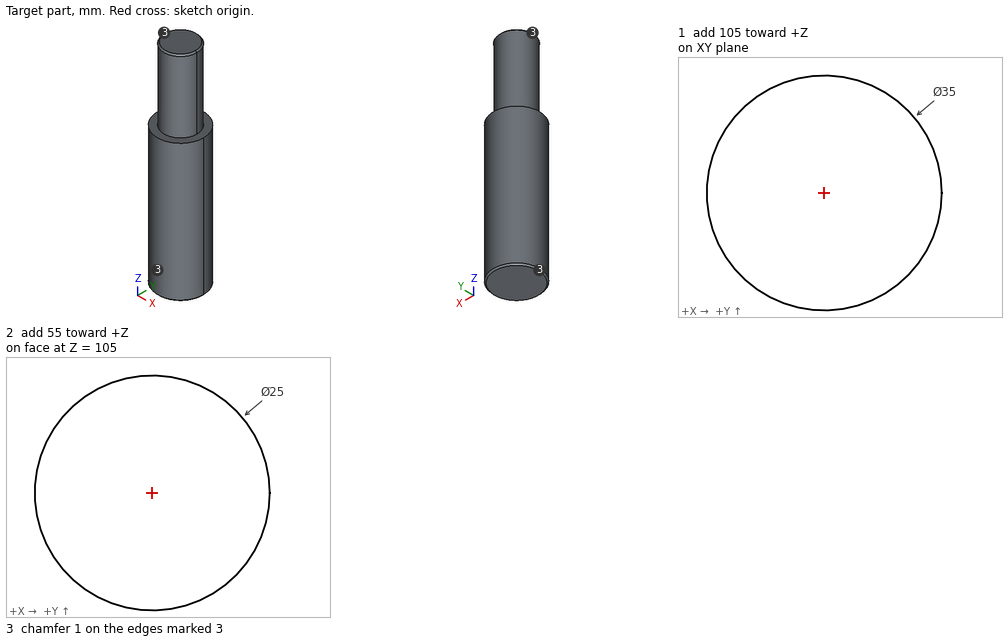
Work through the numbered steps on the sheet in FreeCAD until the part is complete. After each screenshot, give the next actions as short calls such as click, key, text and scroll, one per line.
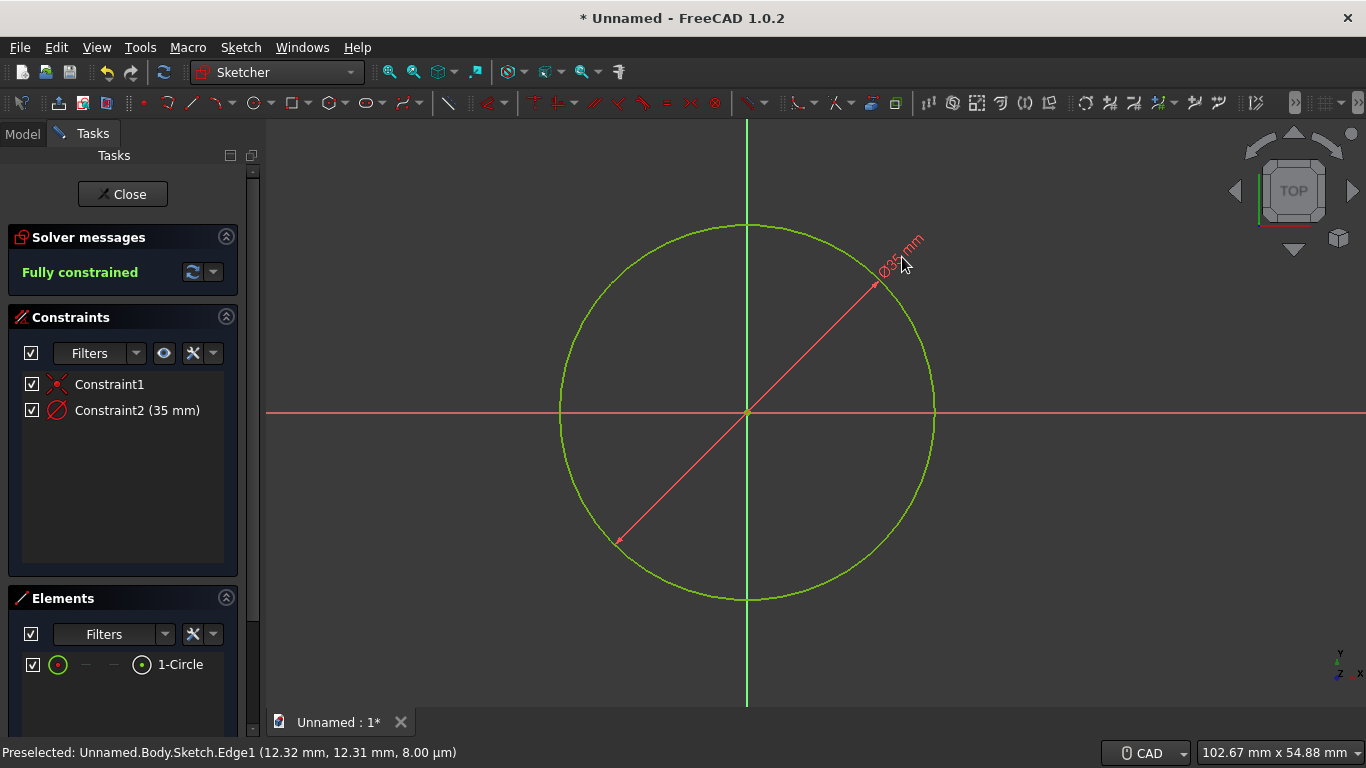
click(123, 194)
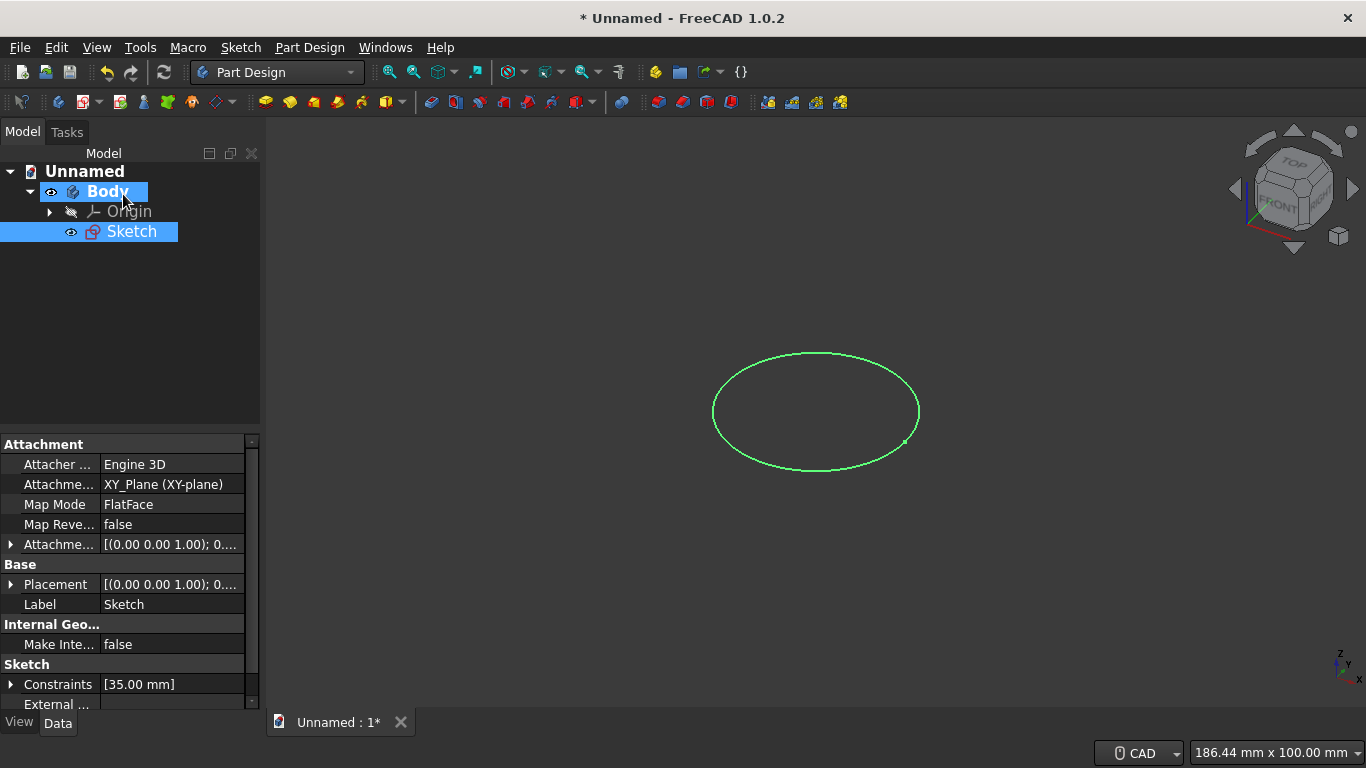
click(266, 102)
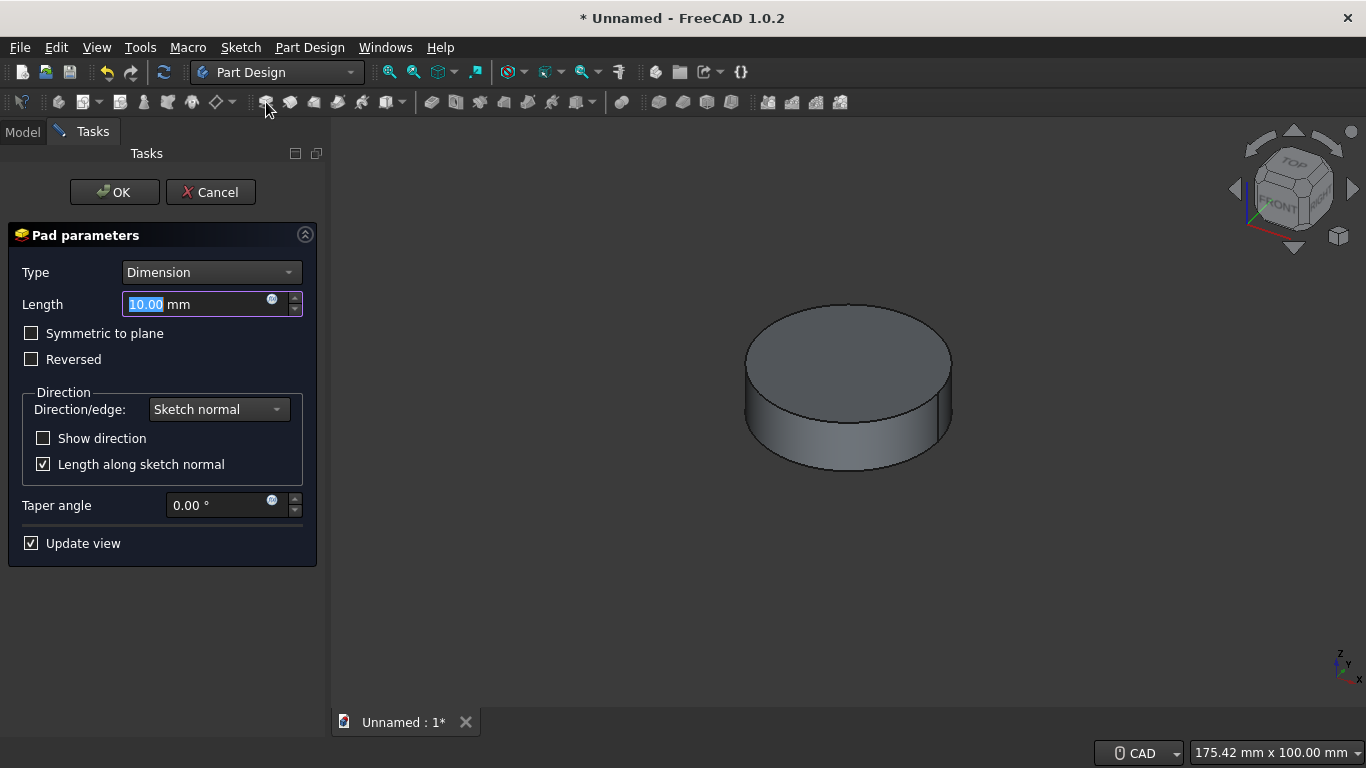
text(105)
key(Tab)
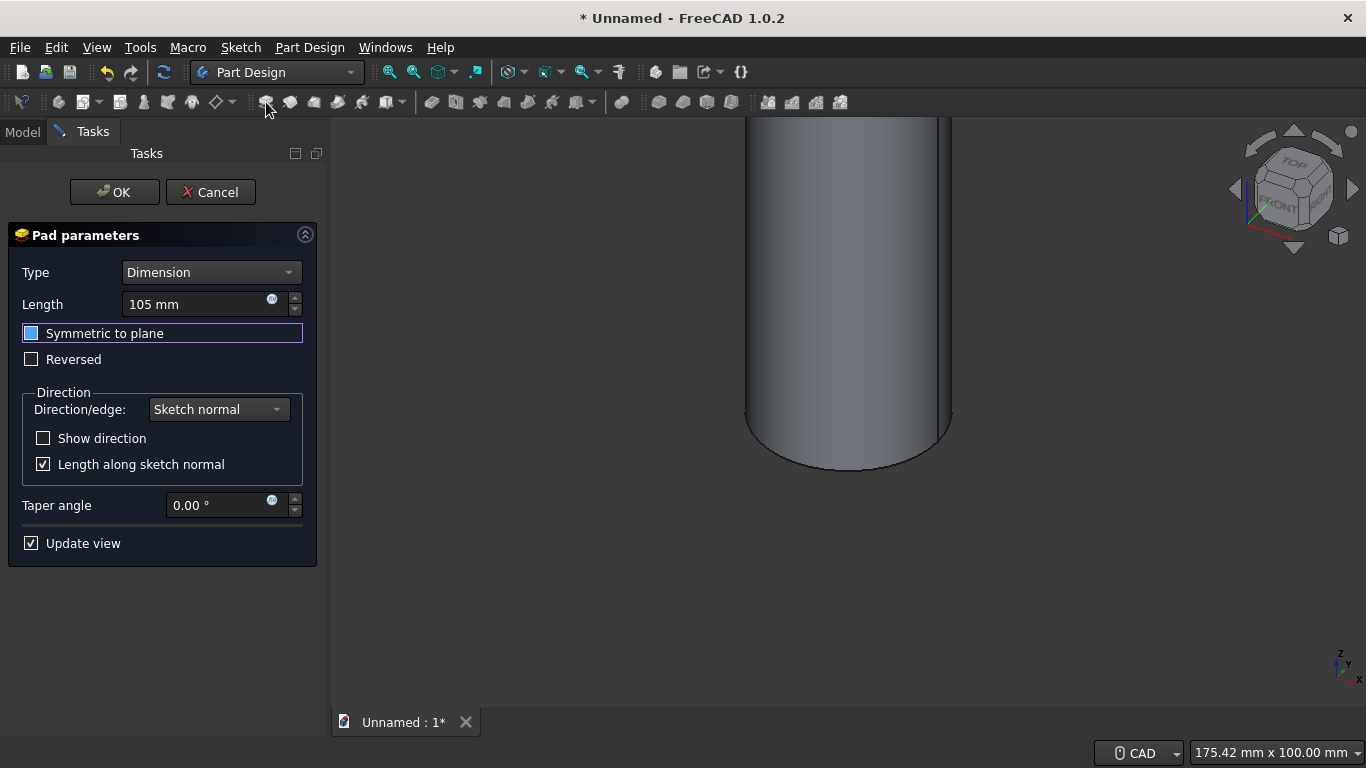
click(115, 192)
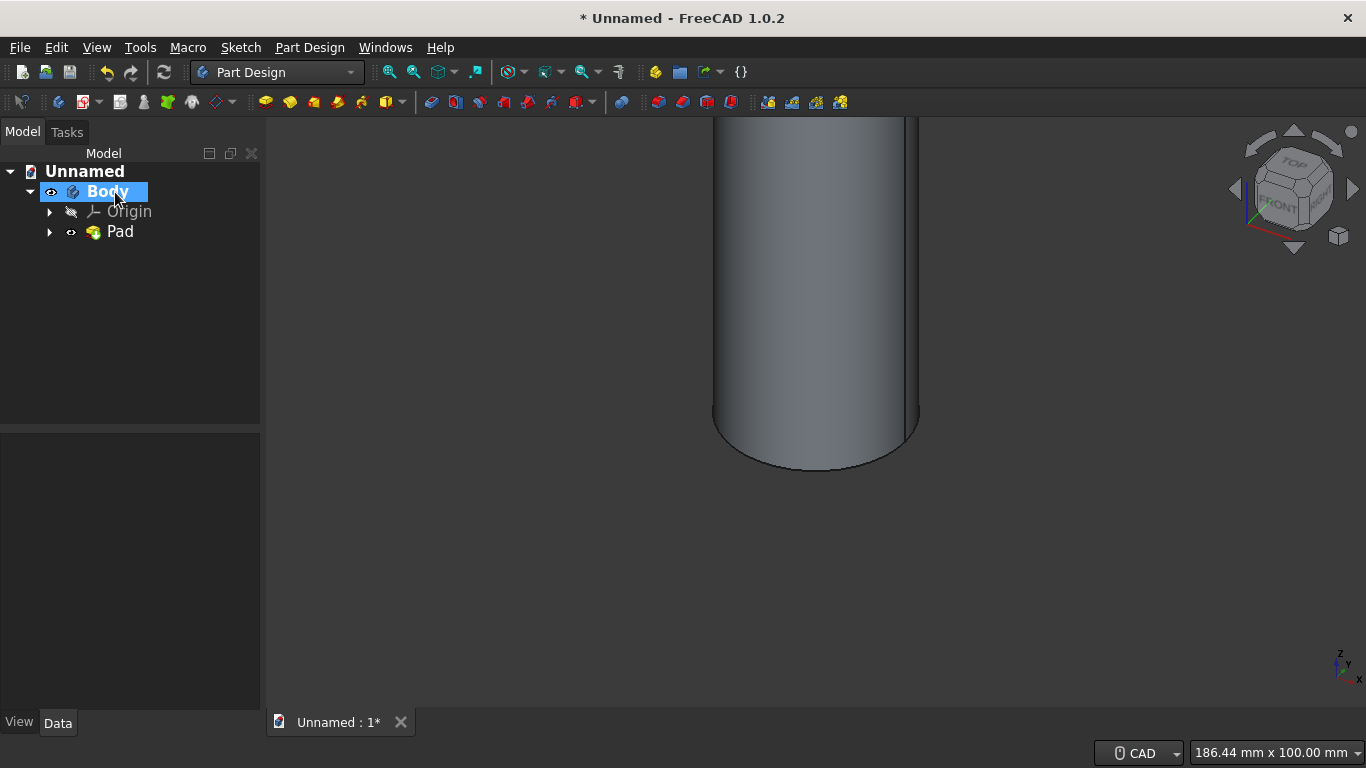
click(390, 72)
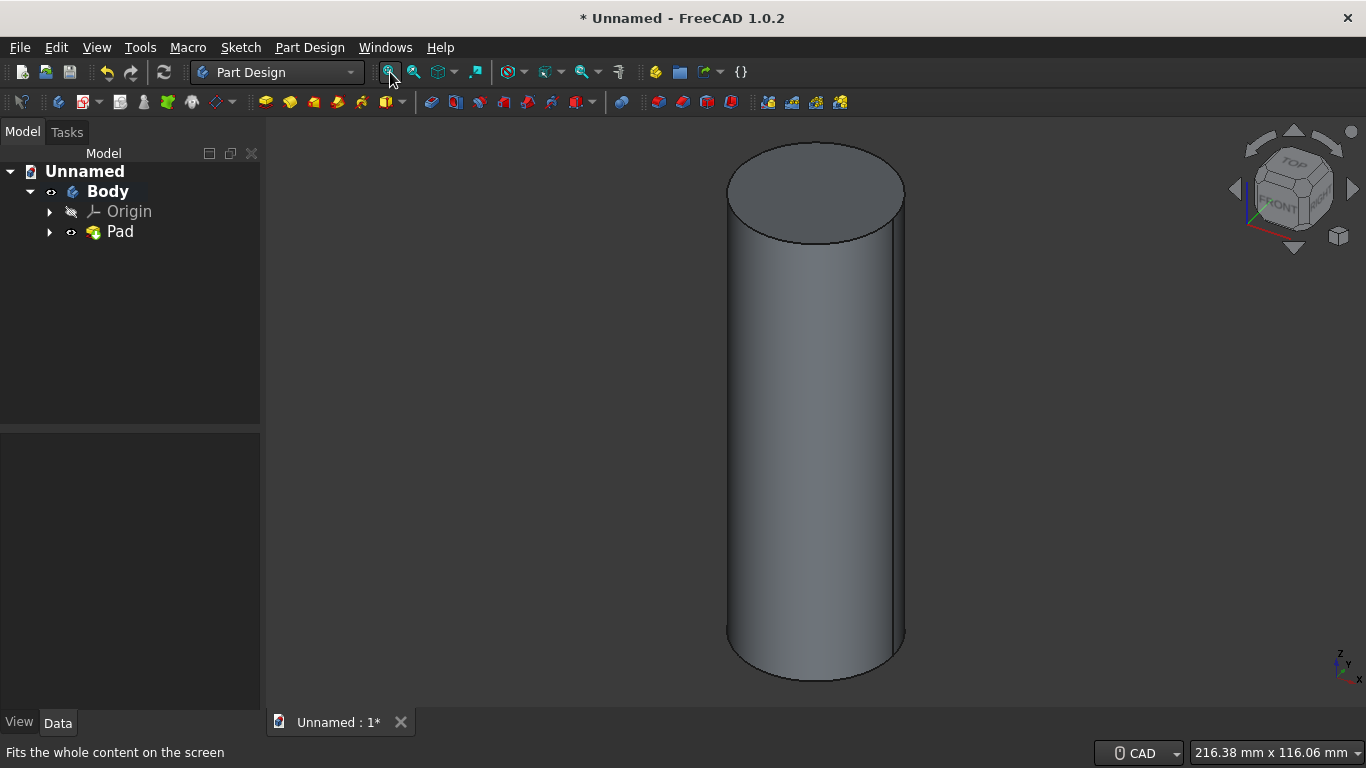
click(816, 192)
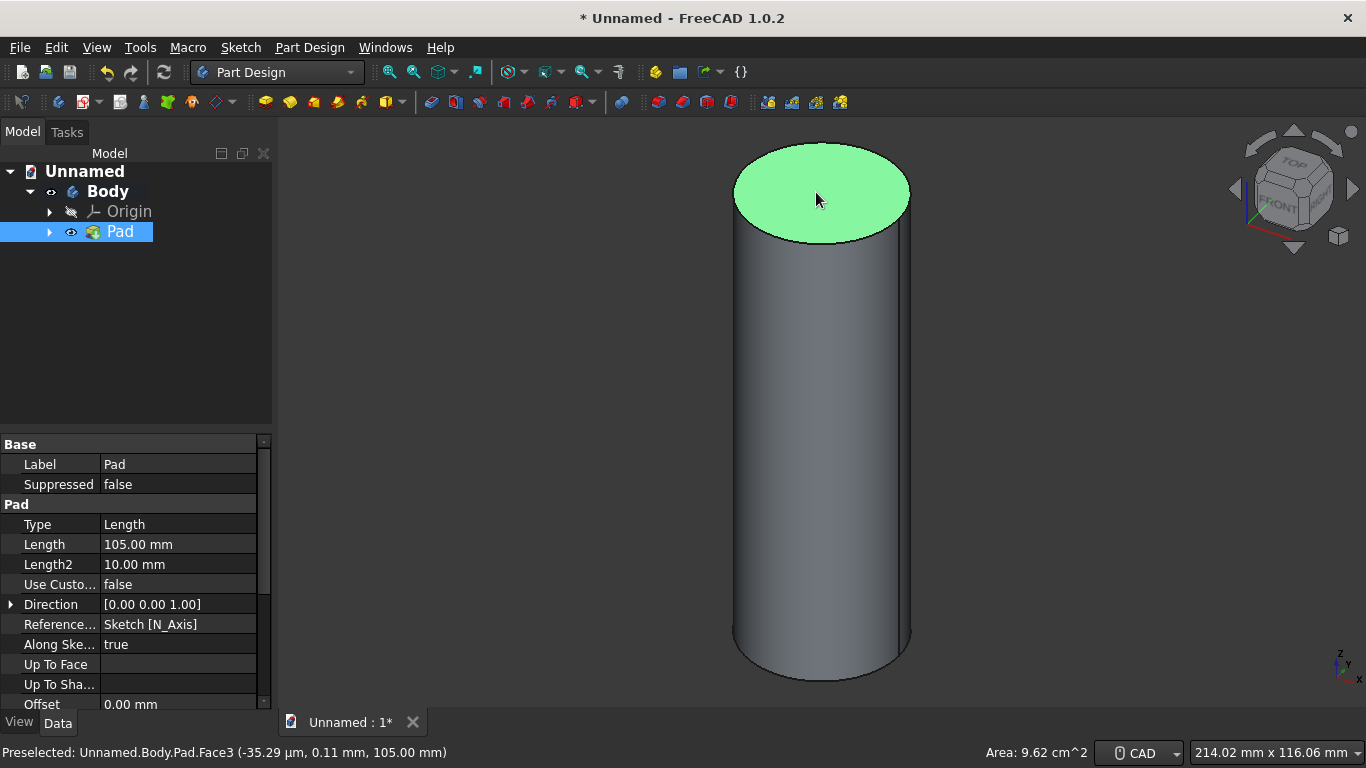
click(84, 102)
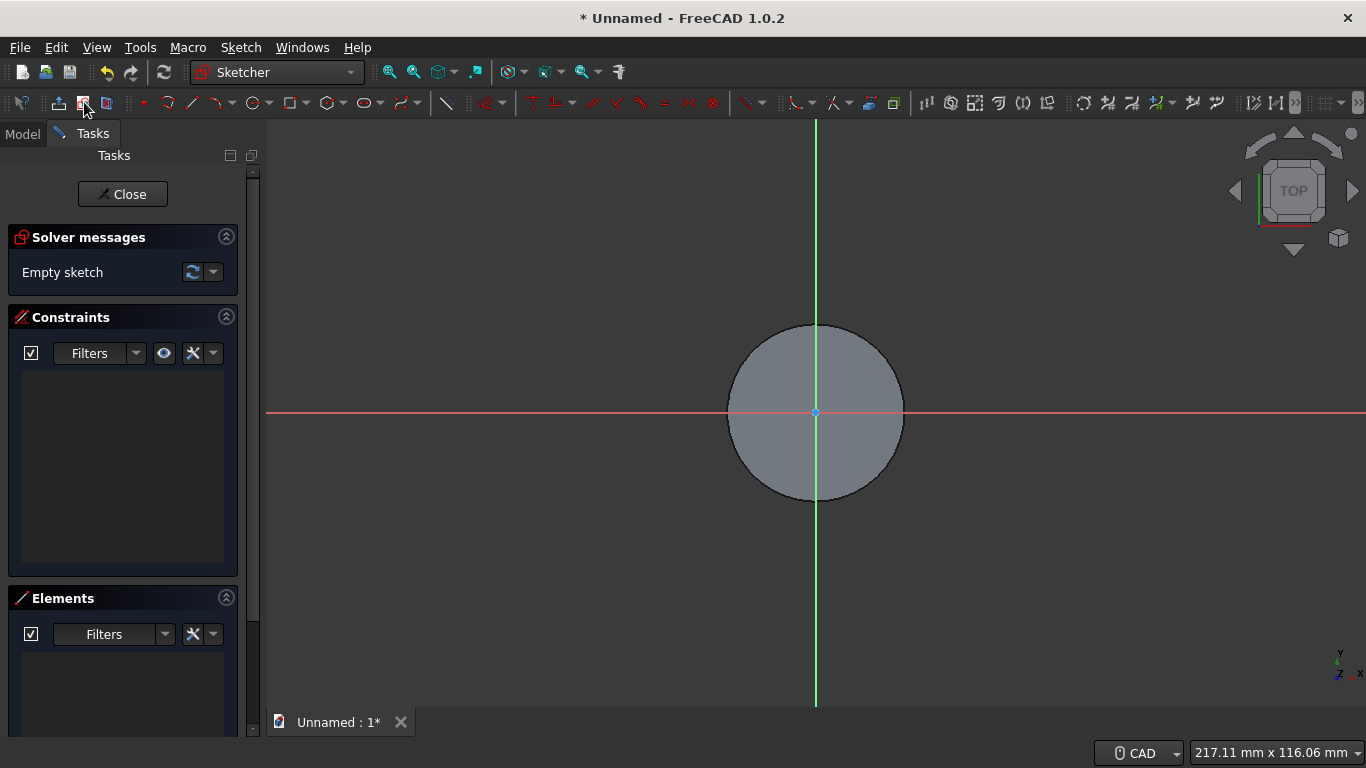
scroll(856, 413, up, 5)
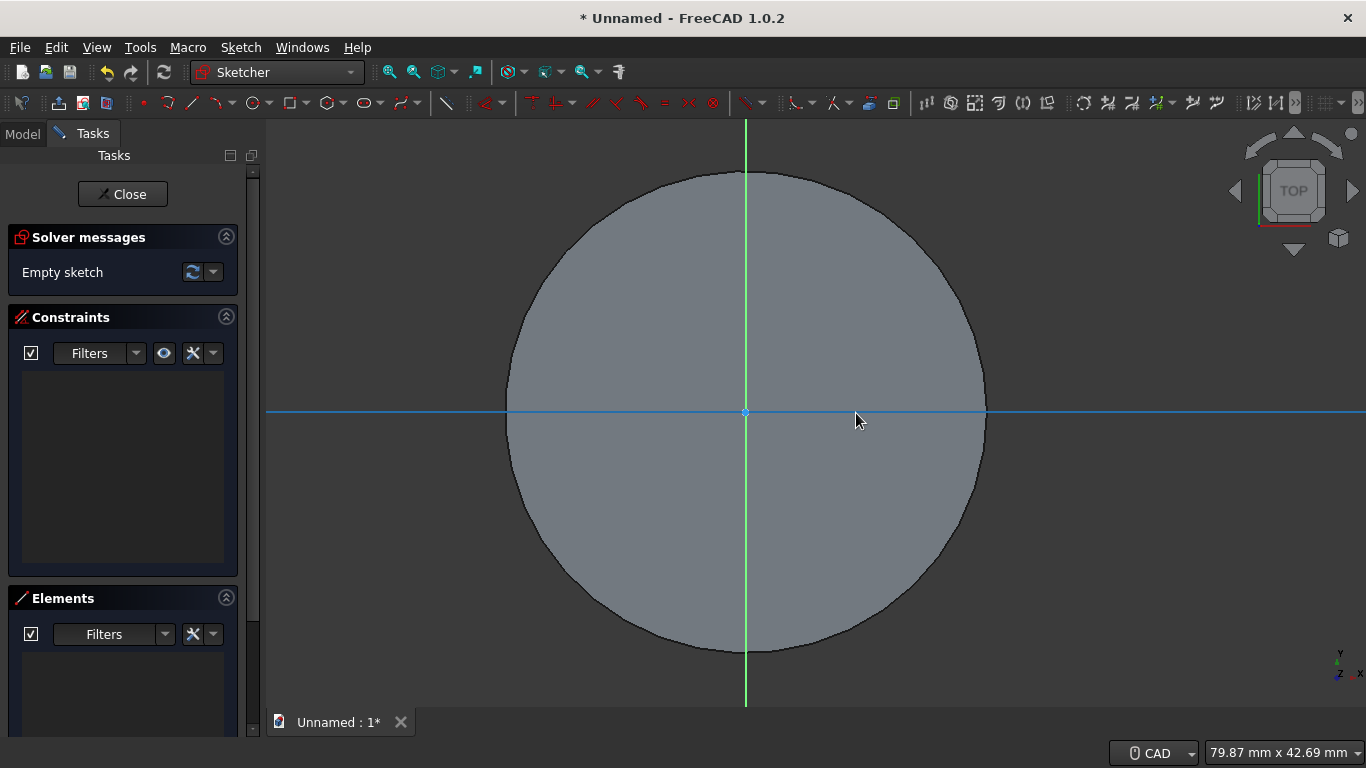
key(g)
key(c)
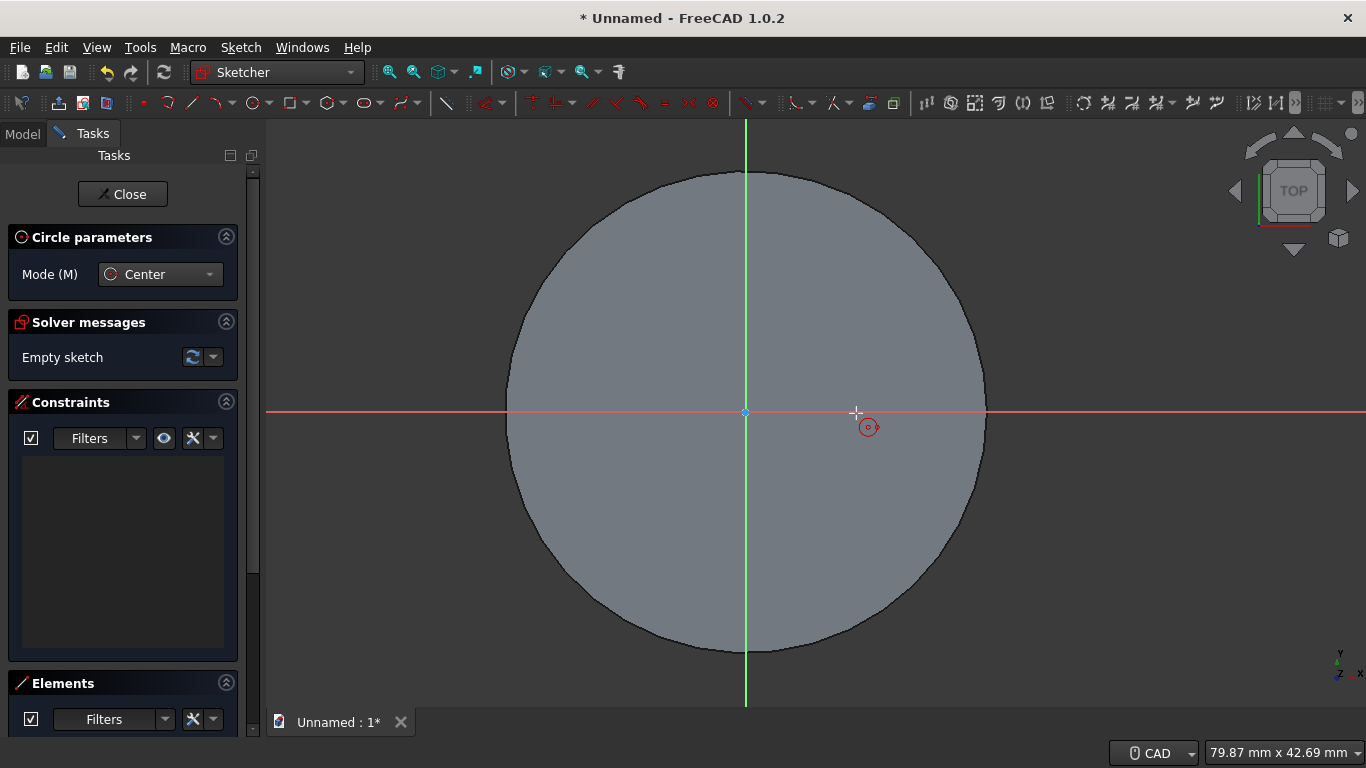
click(746, 412)
click(868, 290)
key(Escape)